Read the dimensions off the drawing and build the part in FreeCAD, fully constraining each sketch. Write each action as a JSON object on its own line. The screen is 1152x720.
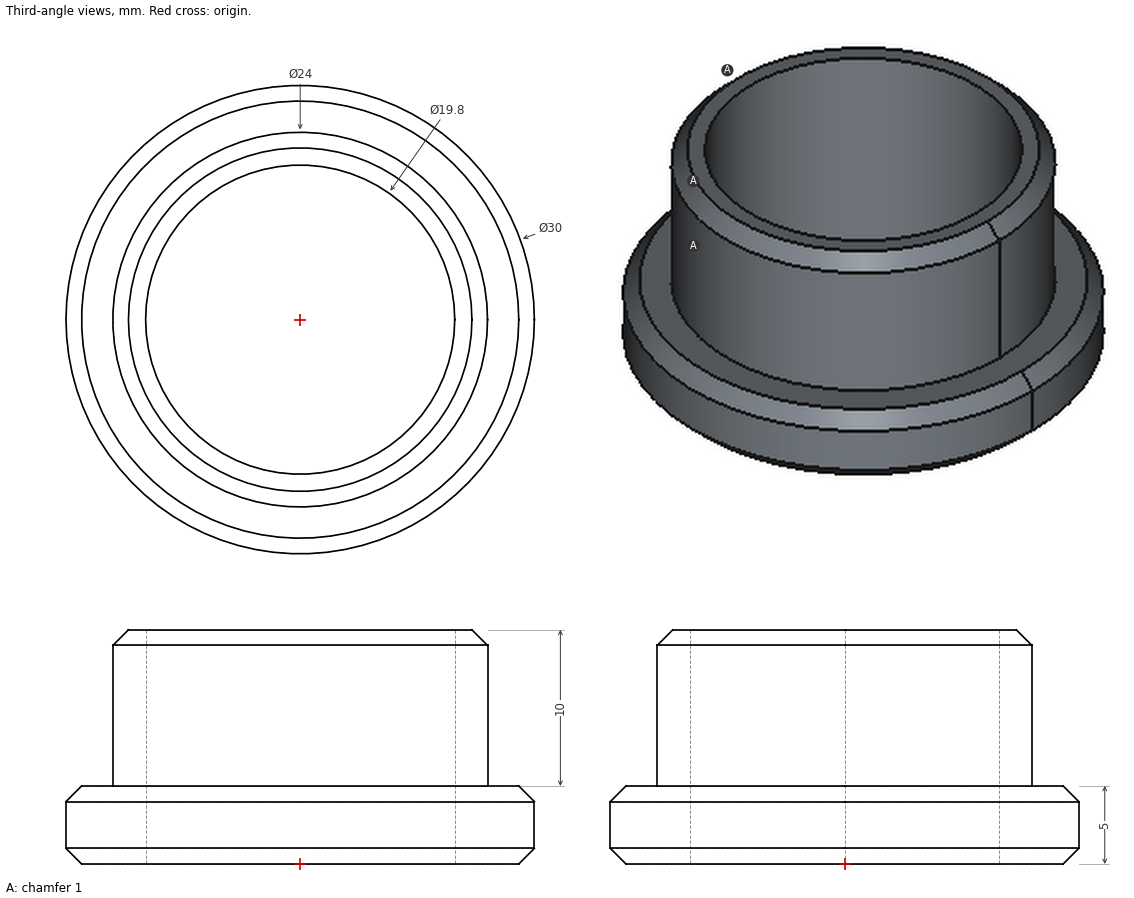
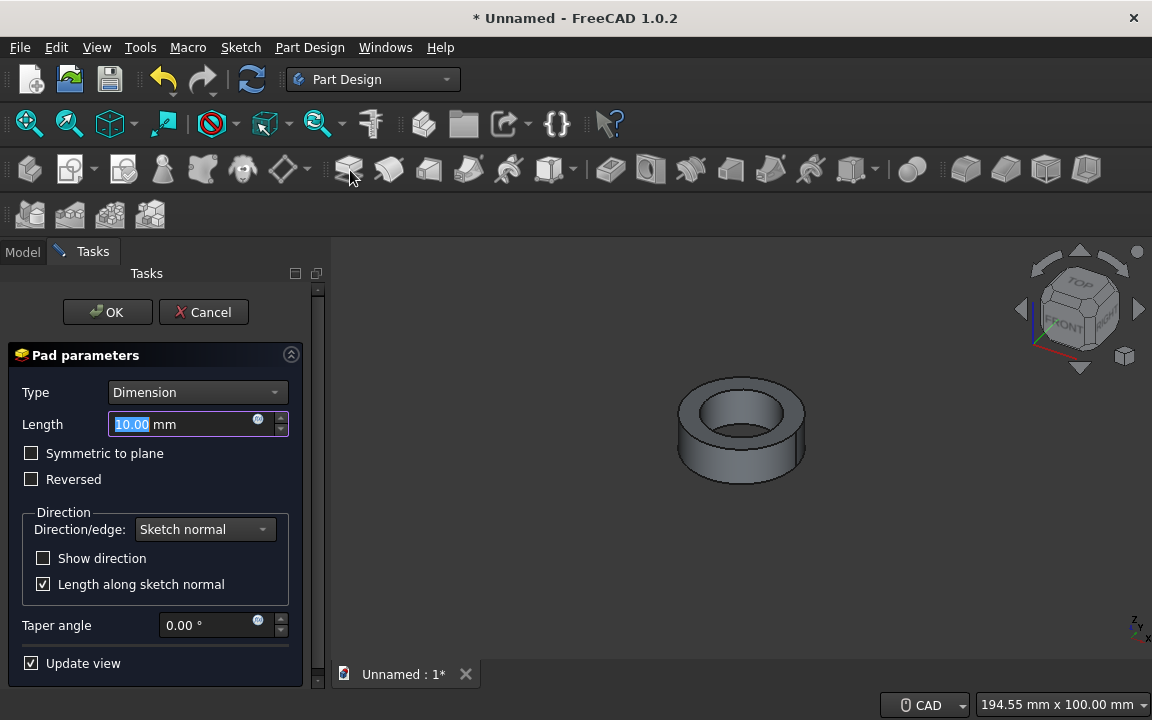
{"action": "type", "text": "5"}
{"action": "key", "text": "Tab"}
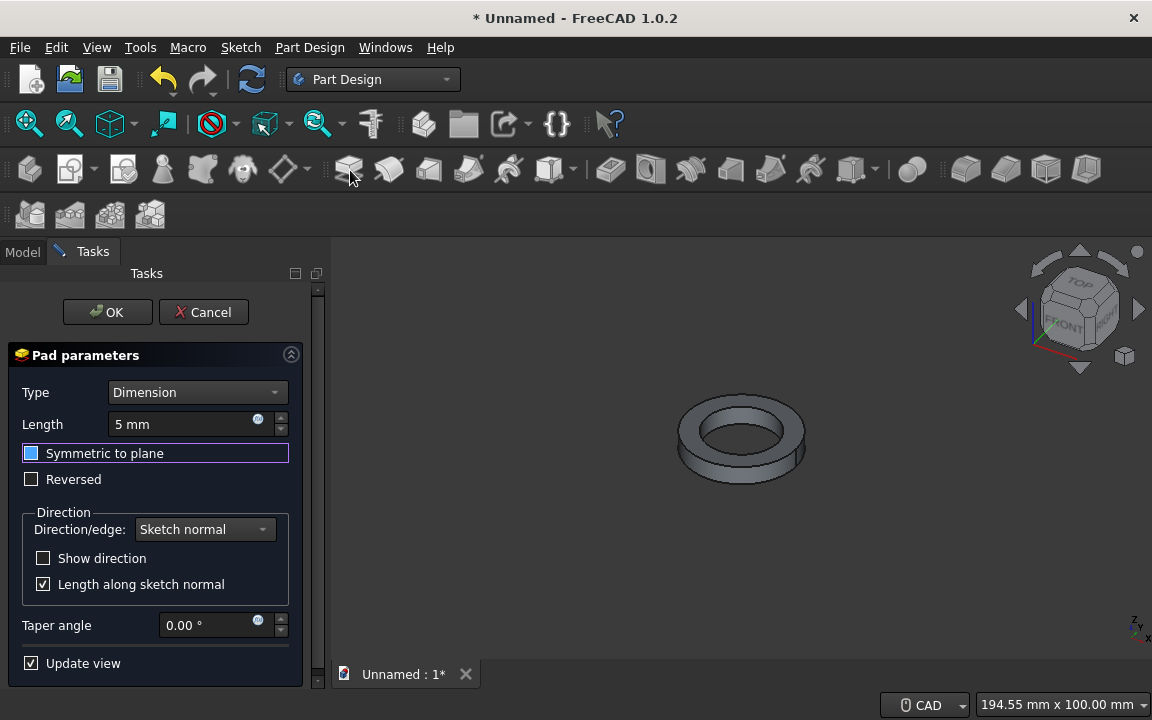
{"action": "left_click", "coordinate": [108, 312]}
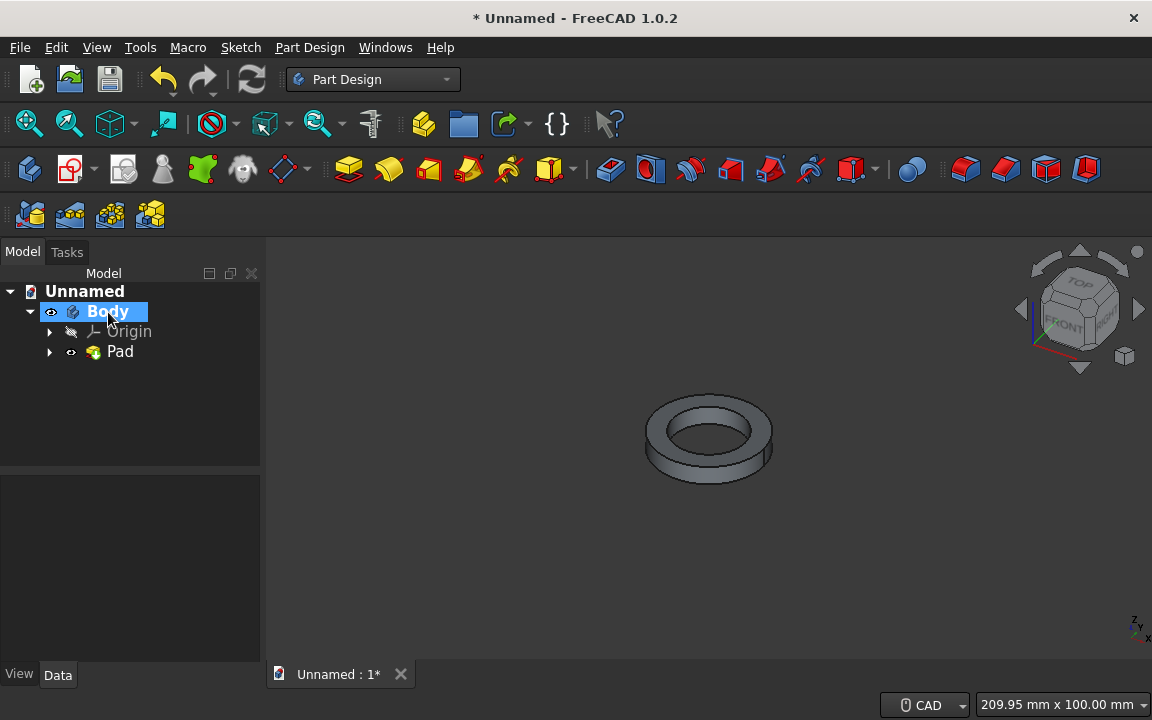
{"action": "left_click", "coordinate": [30, 124]}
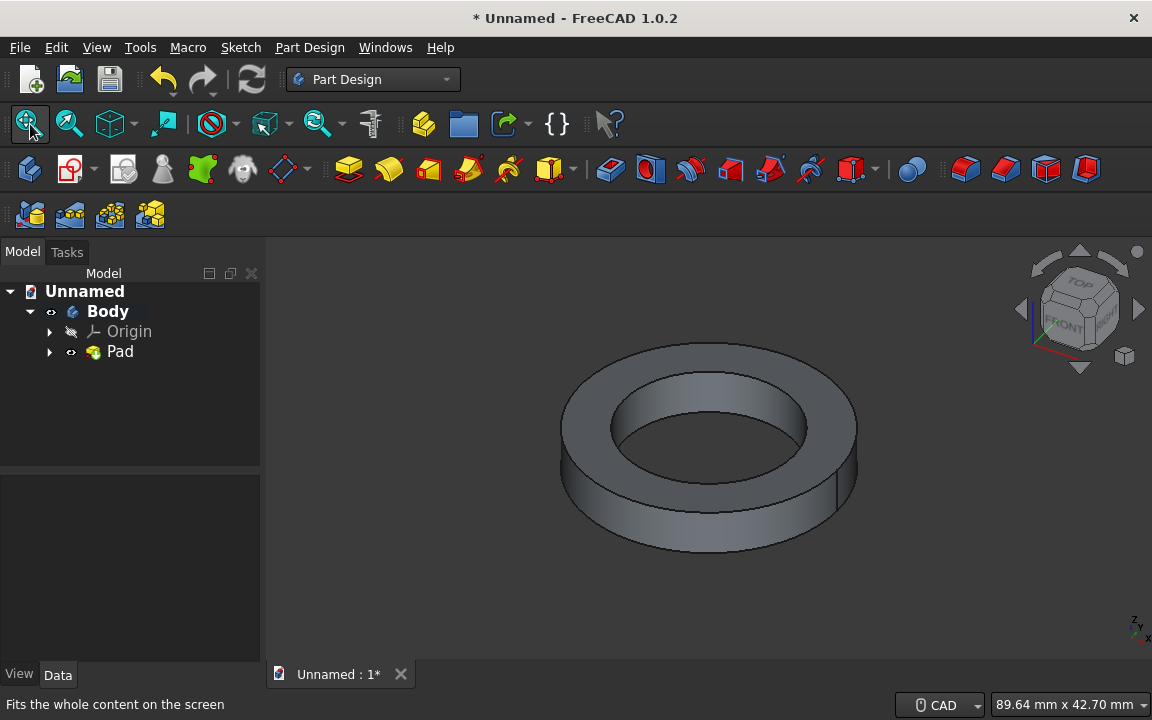
{"action": "left_click", "coordinate": [825, 409]}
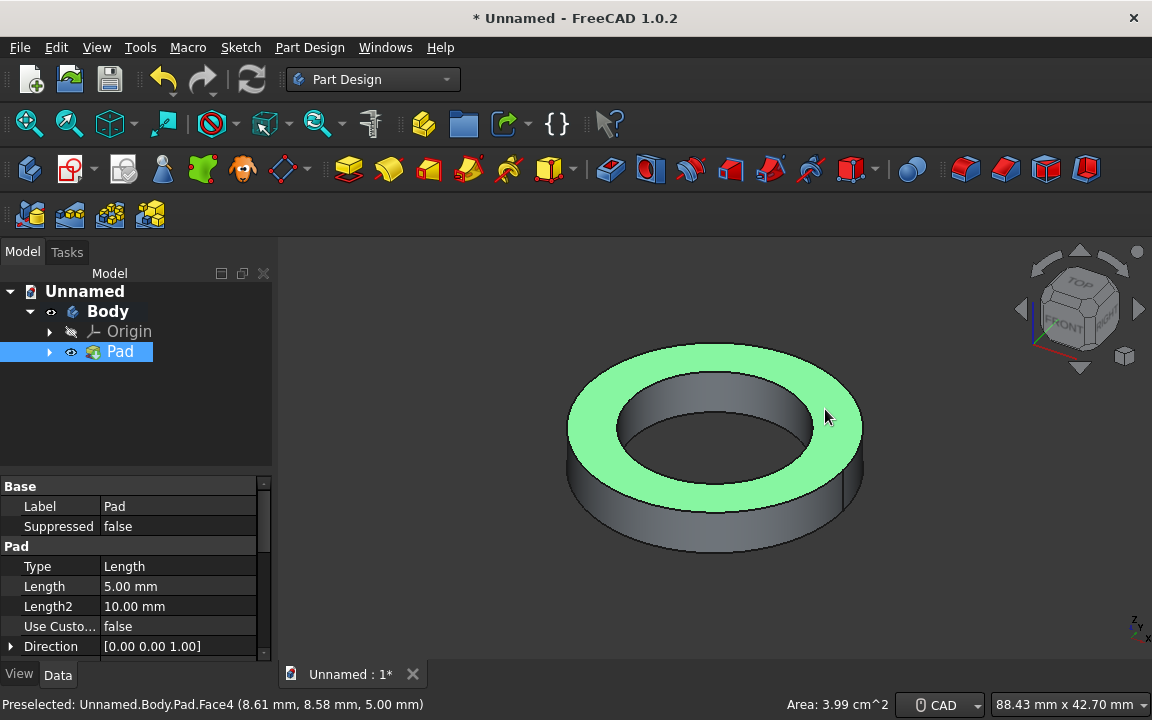
{"action": "left_click", "coordinate": [70, 170]}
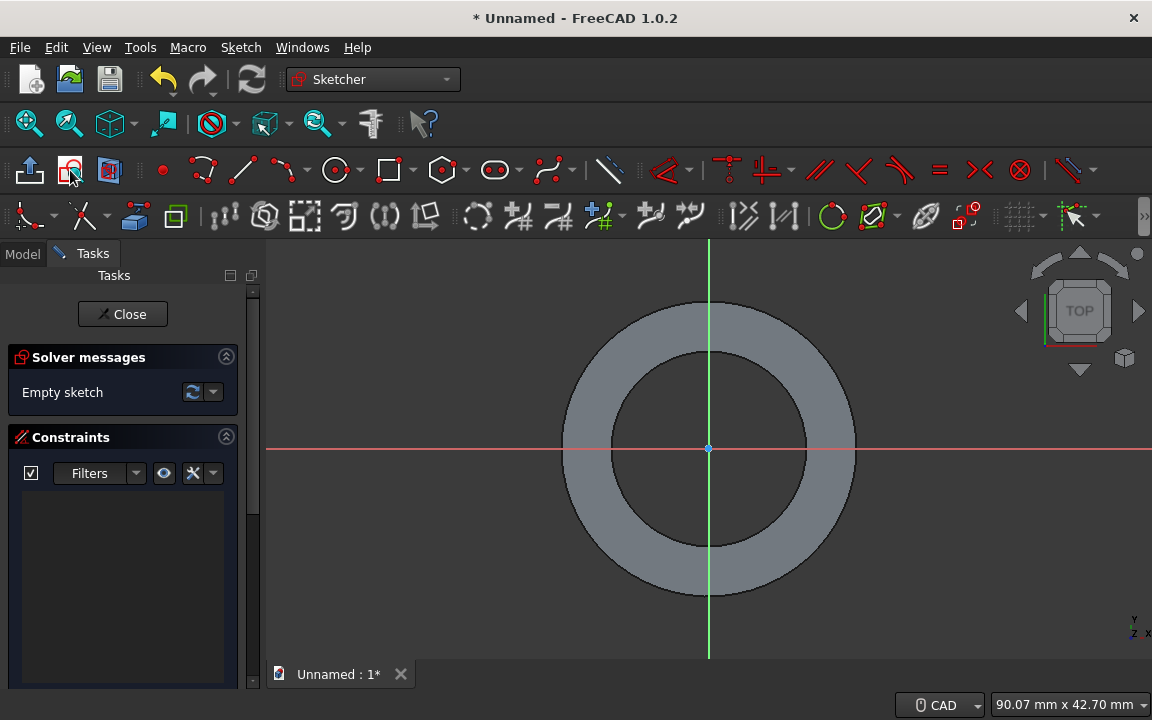
{"action": "left_click", "coordinate": [336, 170]}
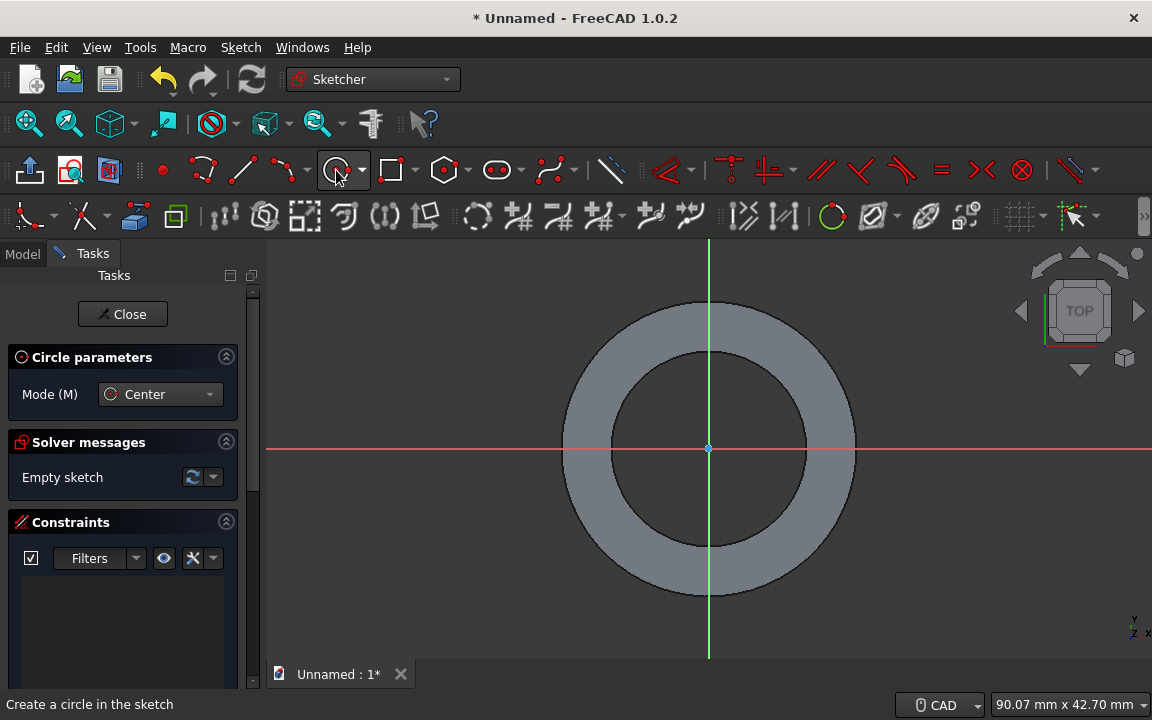
{"action": "left_click", "coordinate": [709, 449]}
{"action": "mouse_move", "coordinate": [792, 366]}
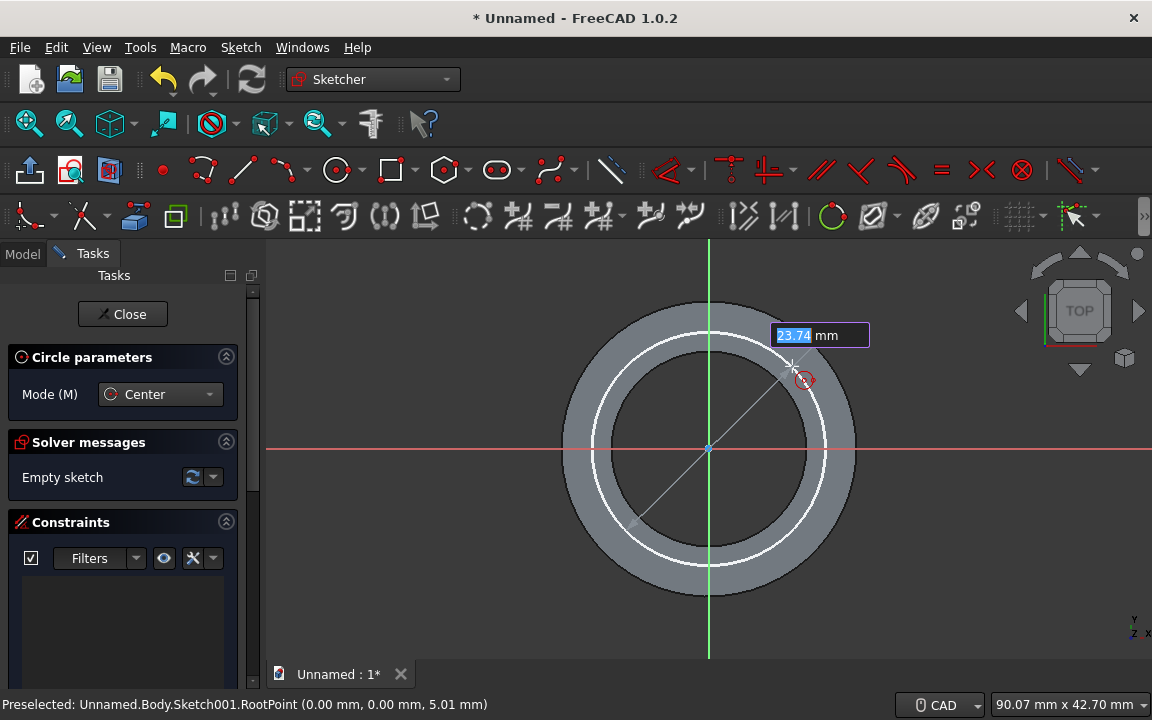
{"action": "type", "text": "24"}
{"action": "key", "text": "Return"}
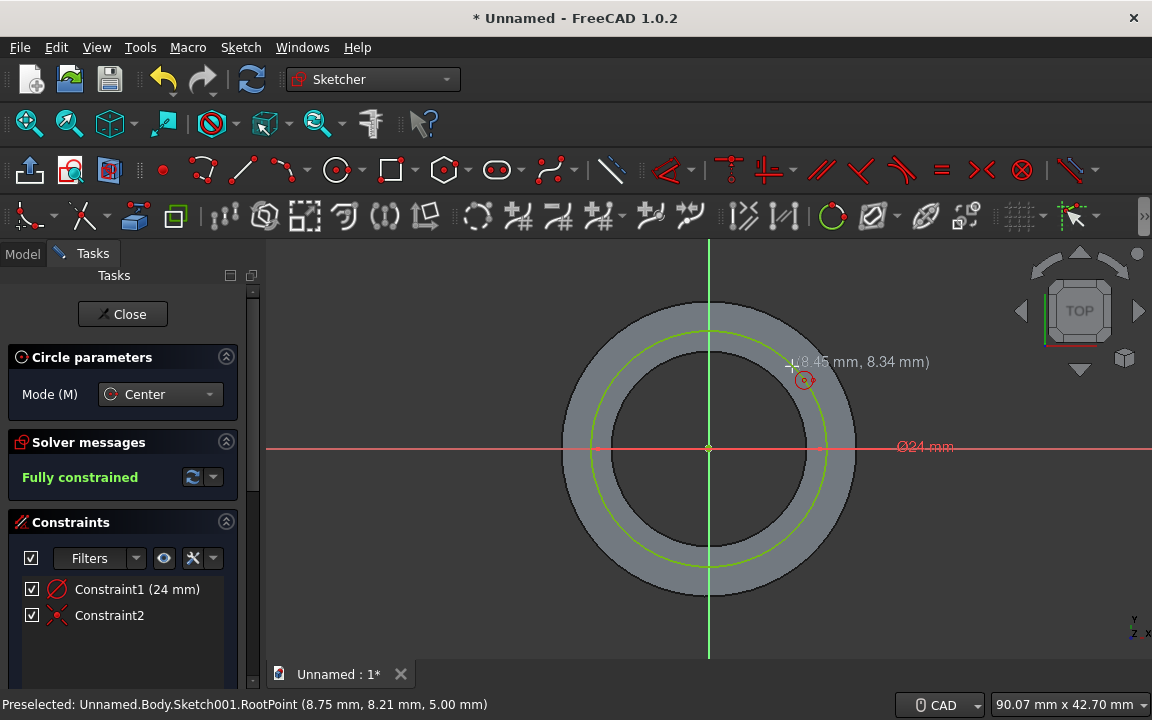
{"action": "left_click", "coordinate": [709, 449]}
{"action": "mouse_move", "coordinate": [778, 380]}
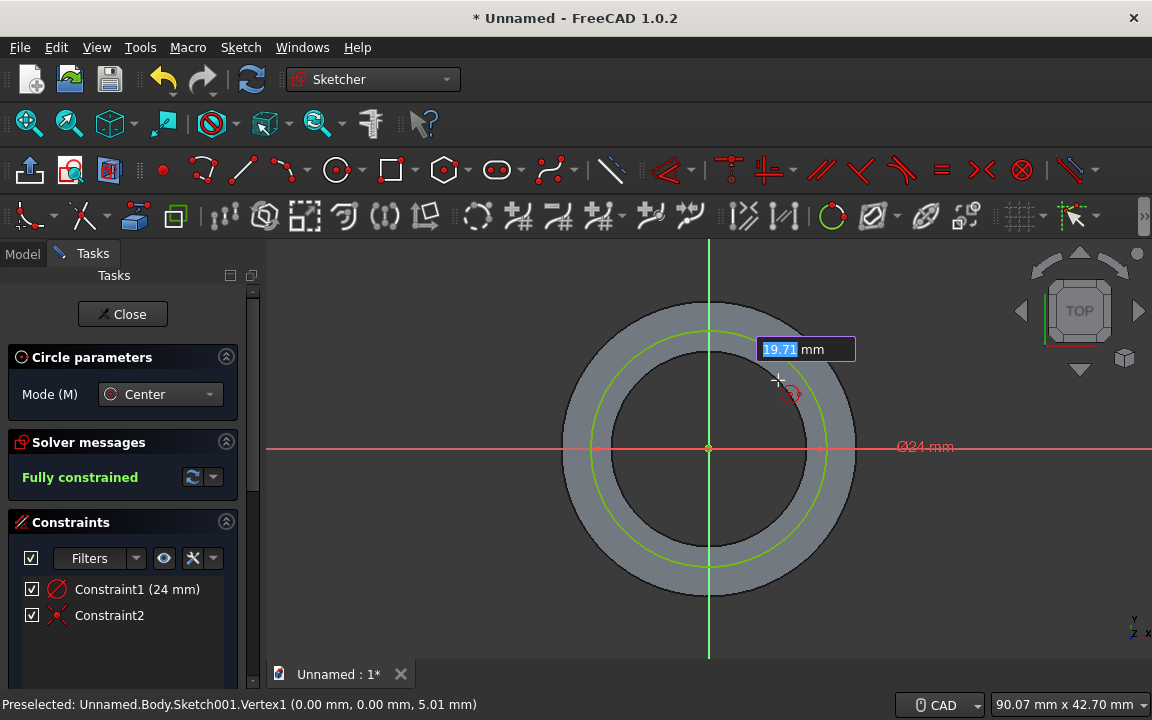
{"action": "type", "text": "19.8"}
{"action": "key", "text": "Return"}
{"action": "key", "text": "Escape"}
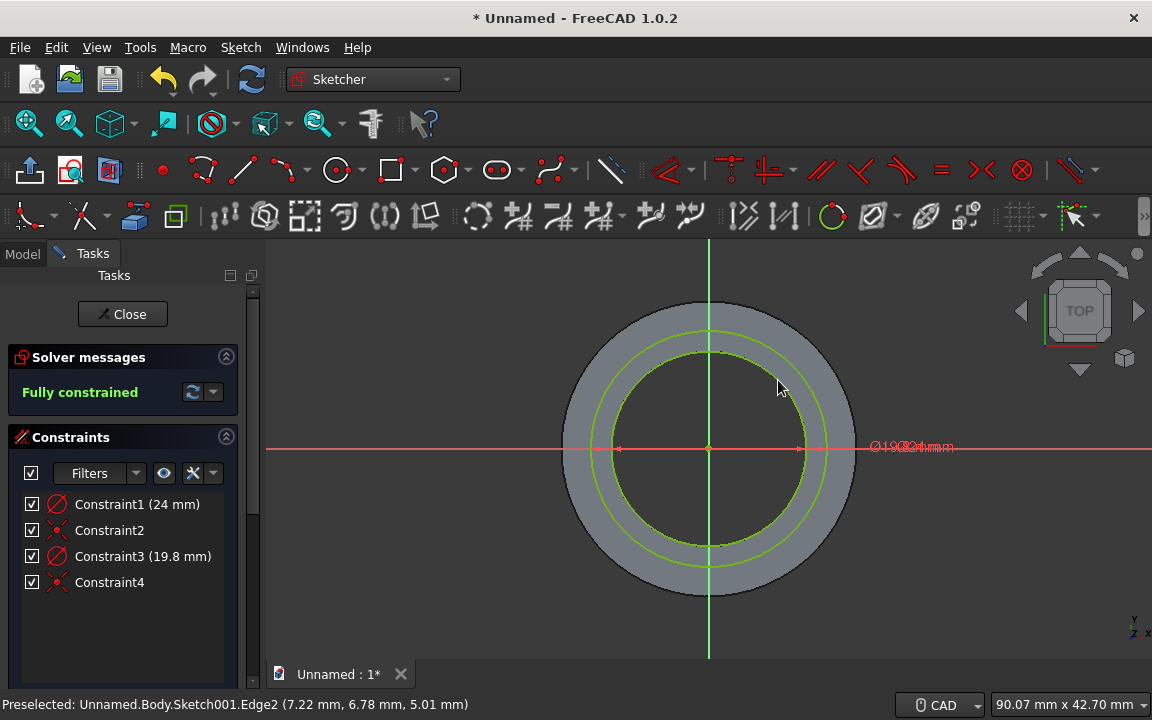
{"action": "left_click", "coordinate": [123, 314]}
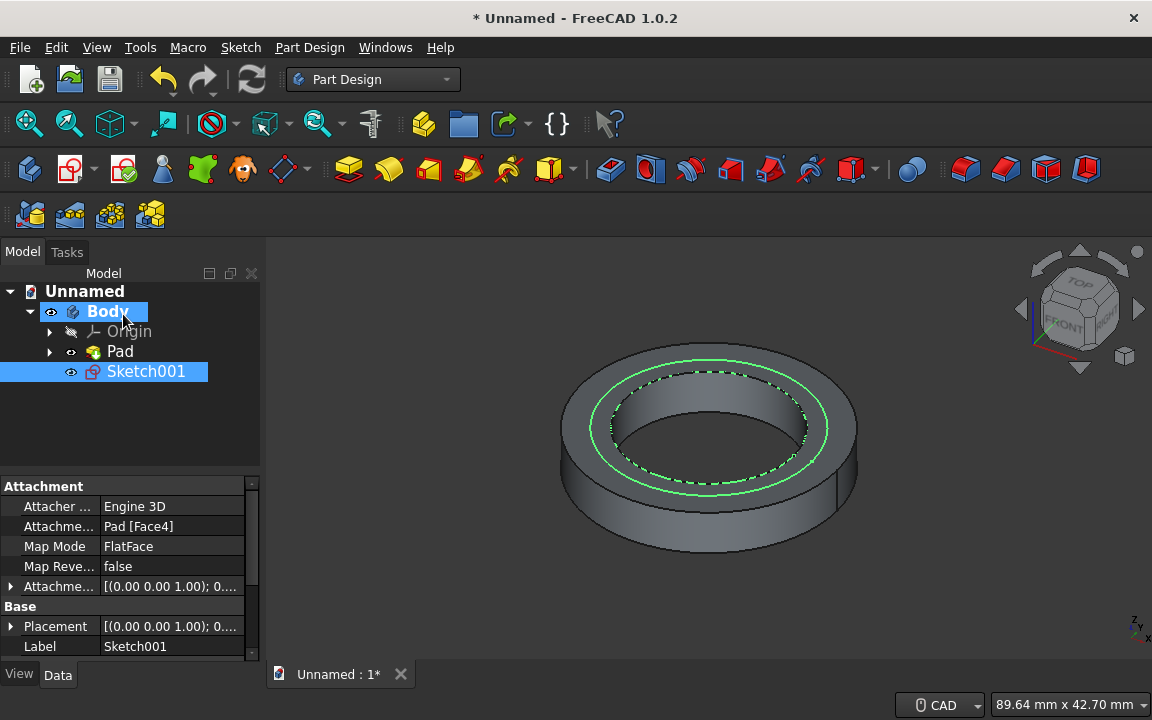
{"action": "left_click", "coordinate": [350, 170]}